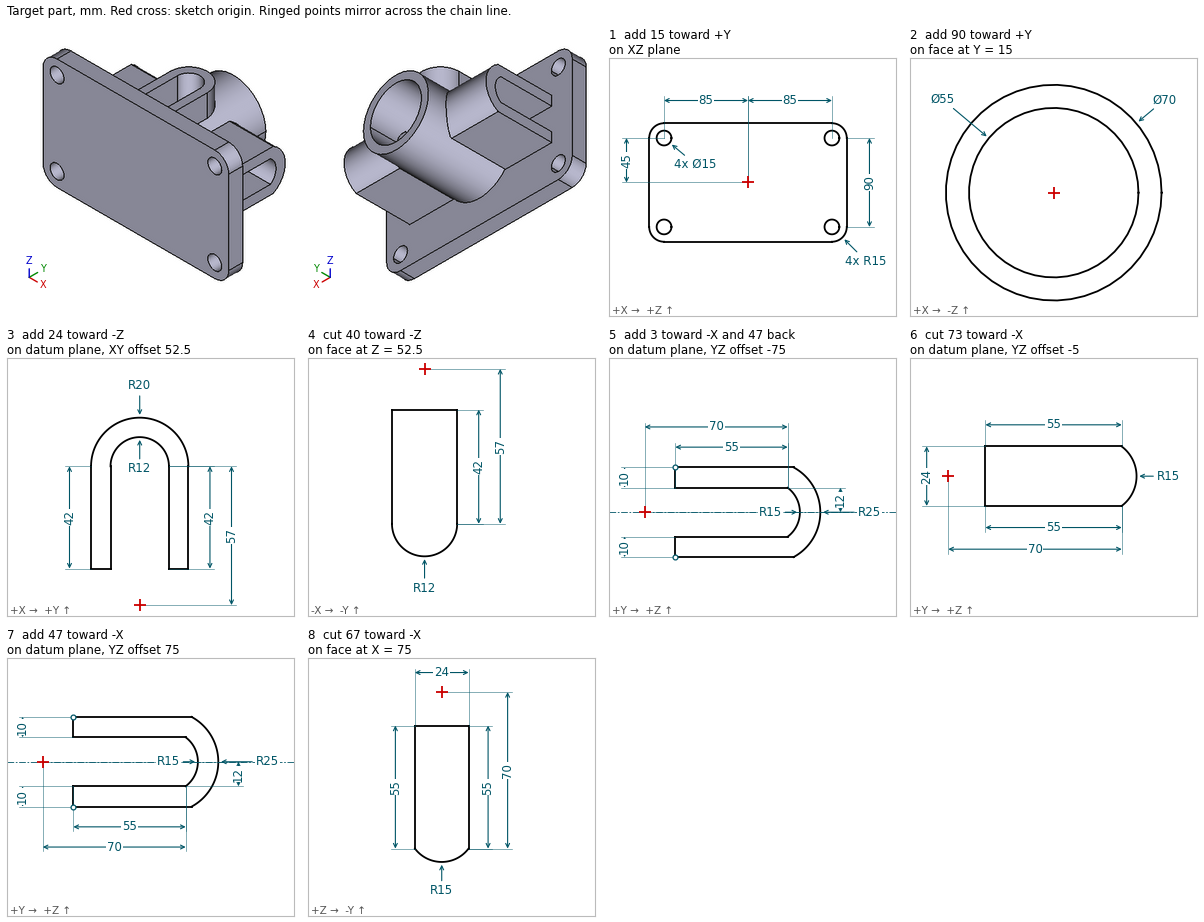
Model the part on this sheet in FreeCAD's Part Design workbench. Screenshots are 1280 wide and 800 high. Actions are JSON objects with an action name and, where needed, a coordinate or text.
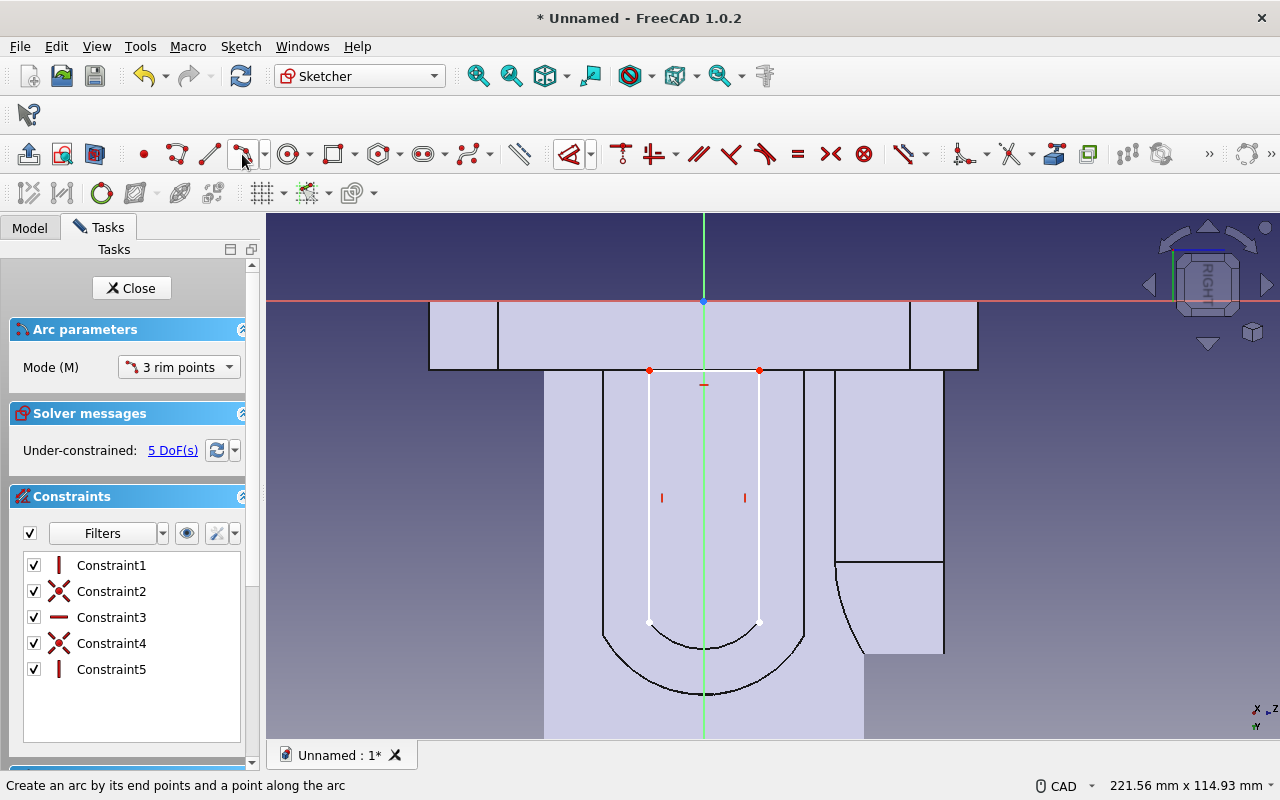
{"action": "left_click", "coordinate": [649, 623]}
{"action": "left_click", "coordinate": [759, 623]}
{"action": "left_click", "coordinate": [679, 645]}
{"action": "key", "text": "Escape"}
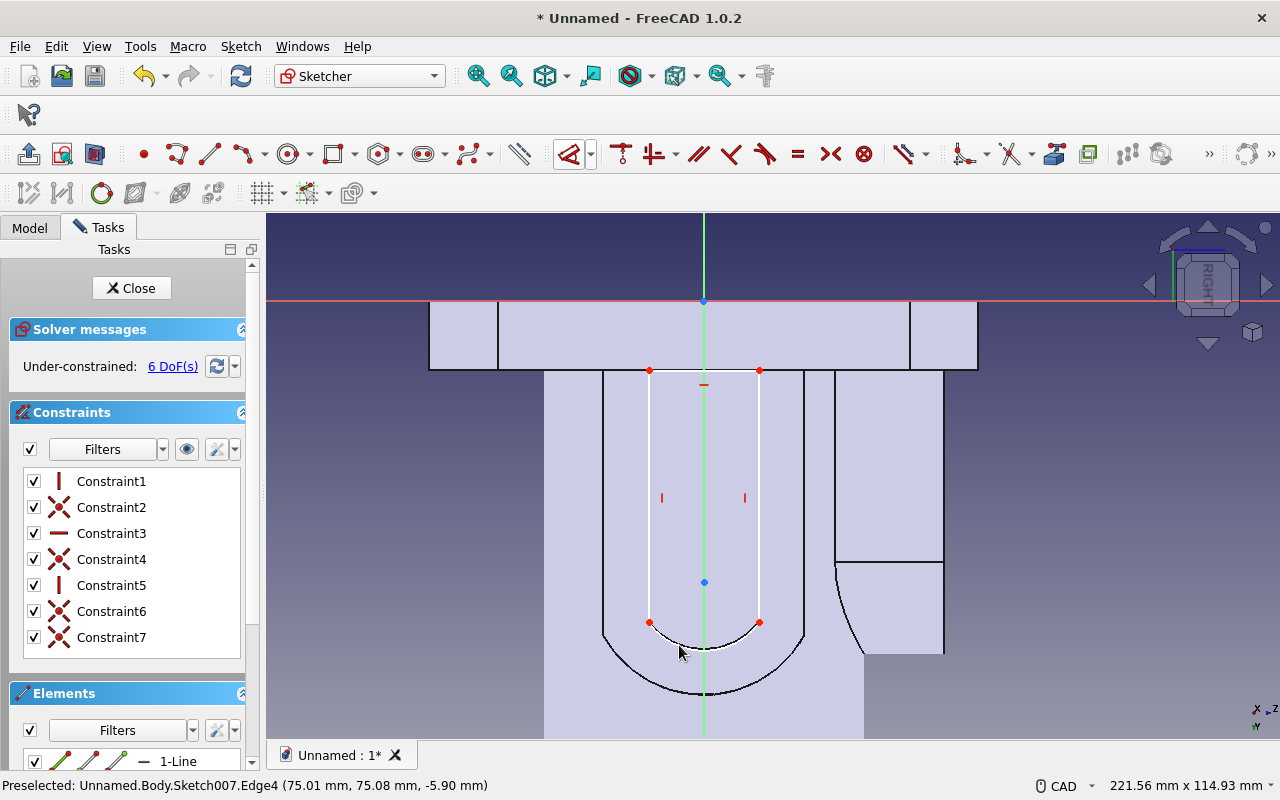
{"action": "left_click", "coordinate": [704, 582]}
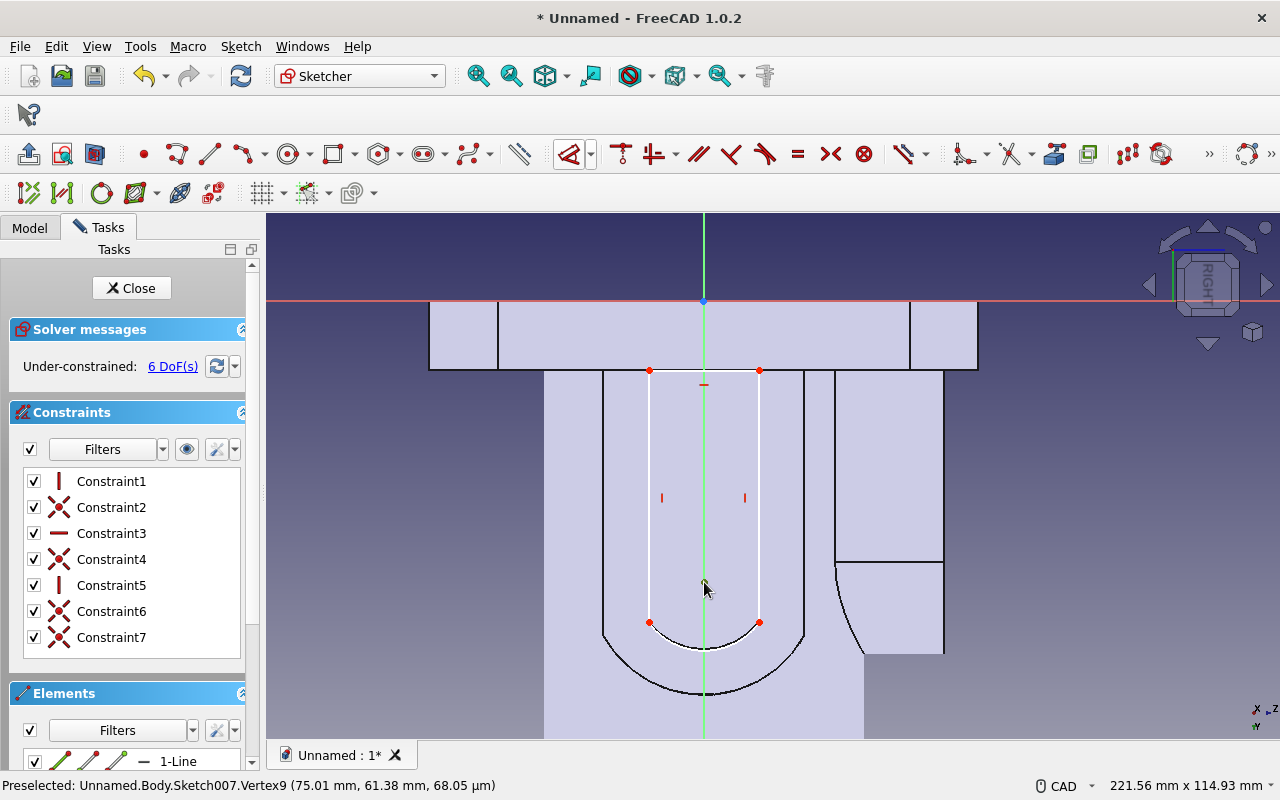
{"action": "left_click", "coordinate": [704, 610]}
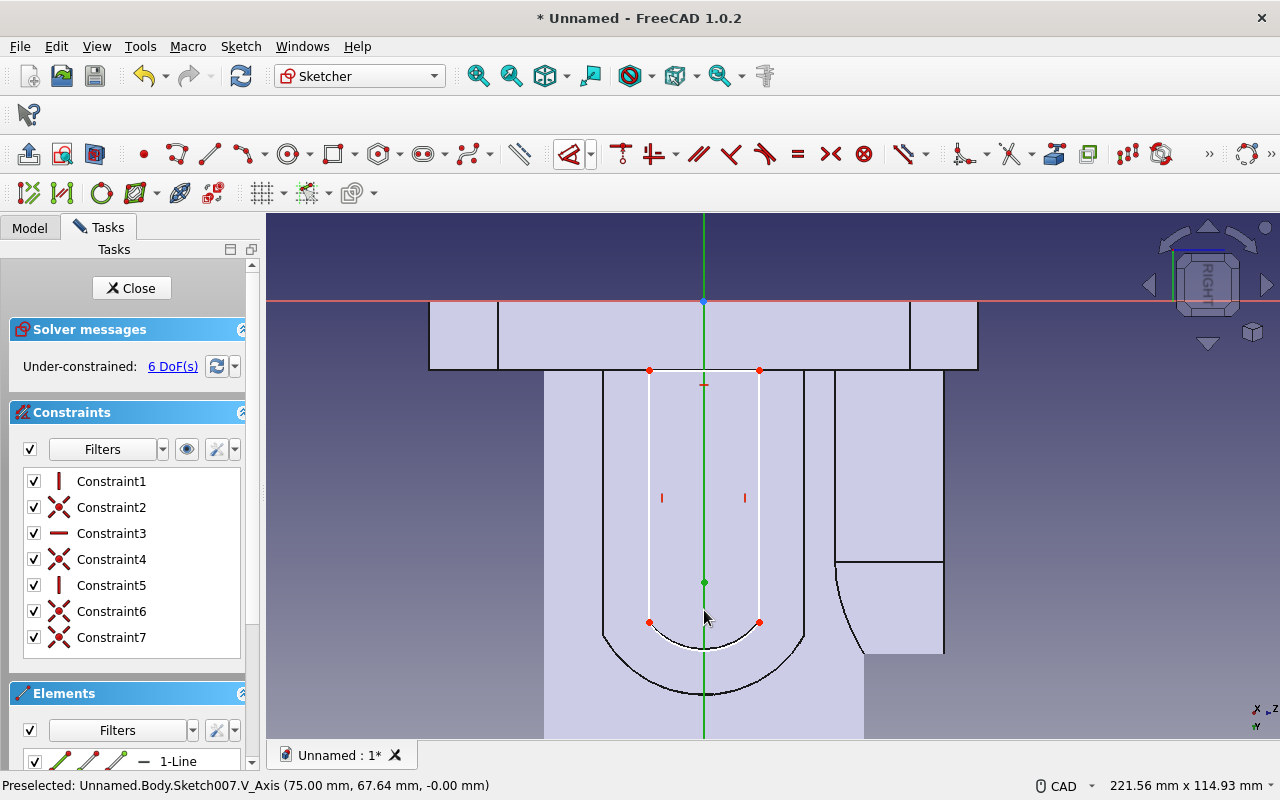
{"action": "key", "text": "c"}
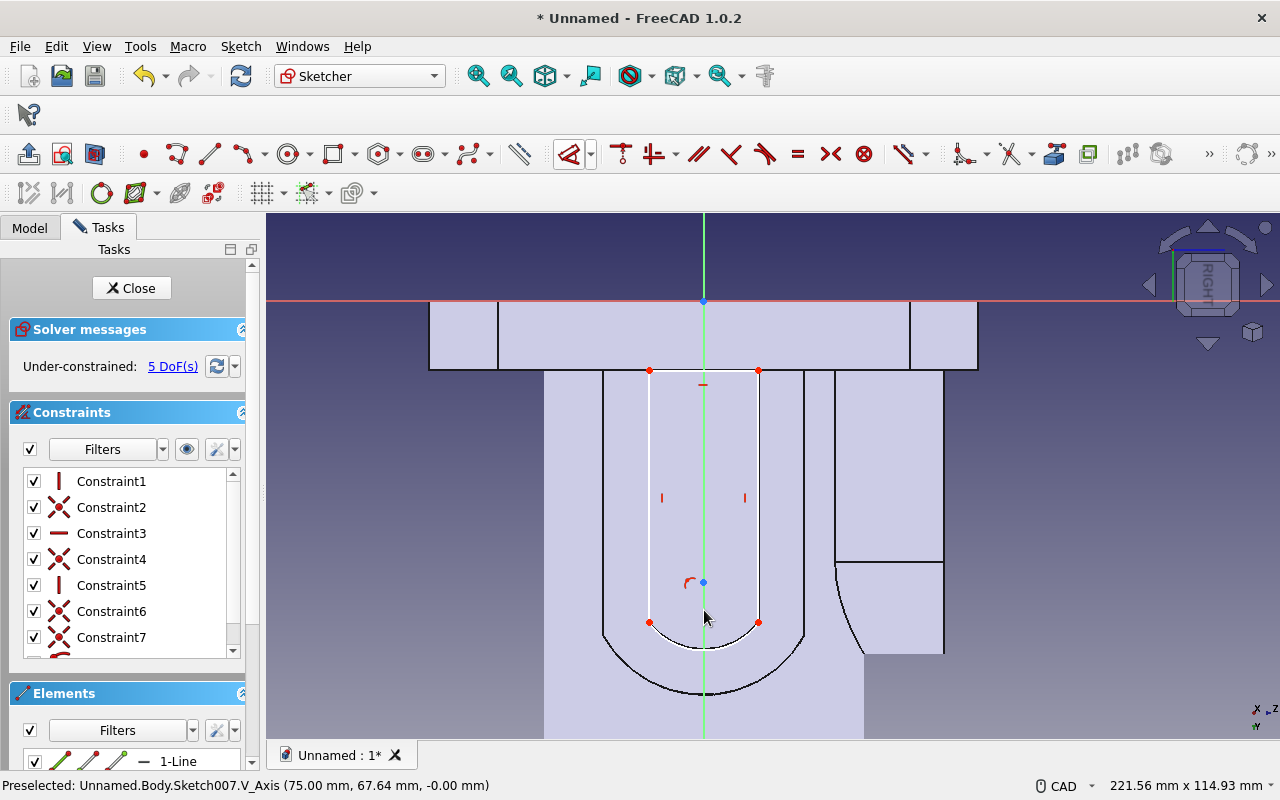
{"action": "left_click", "coordinate": [679, 646]}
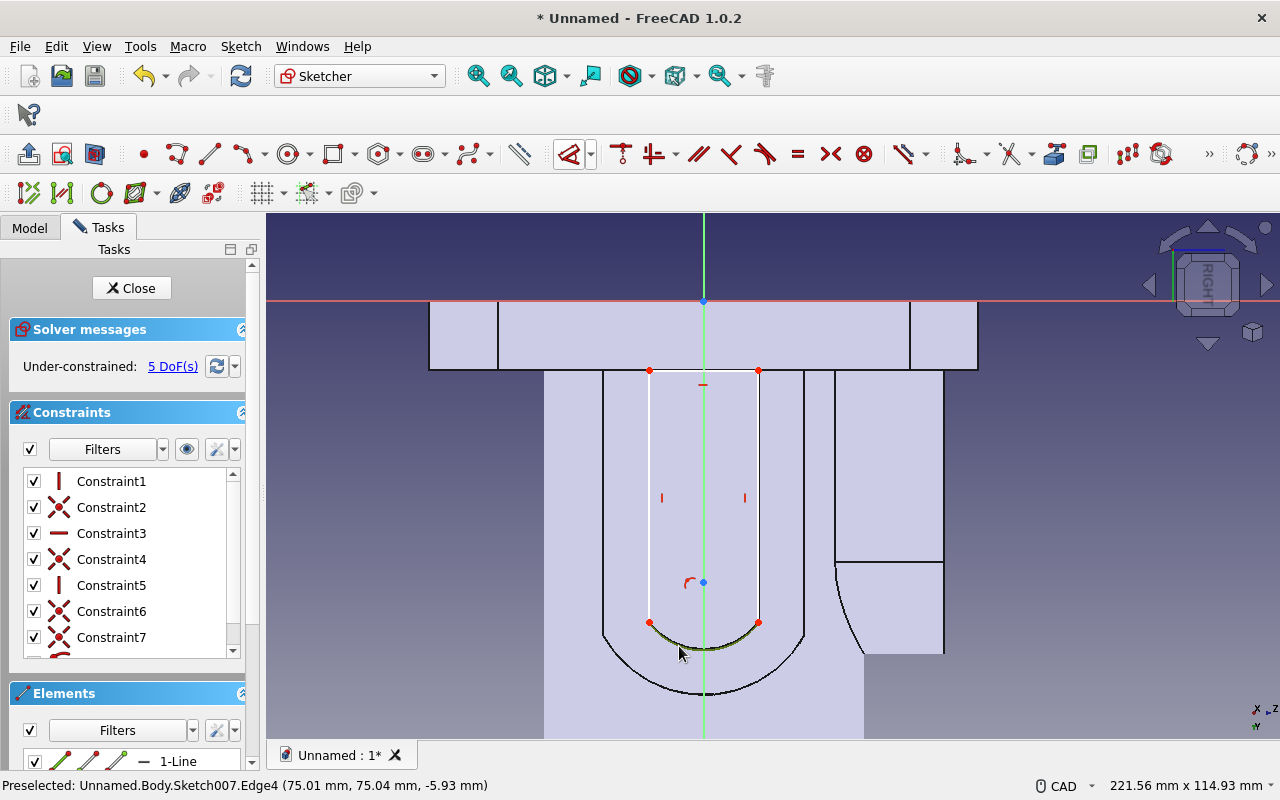
{"action": "key", "text": "k r"}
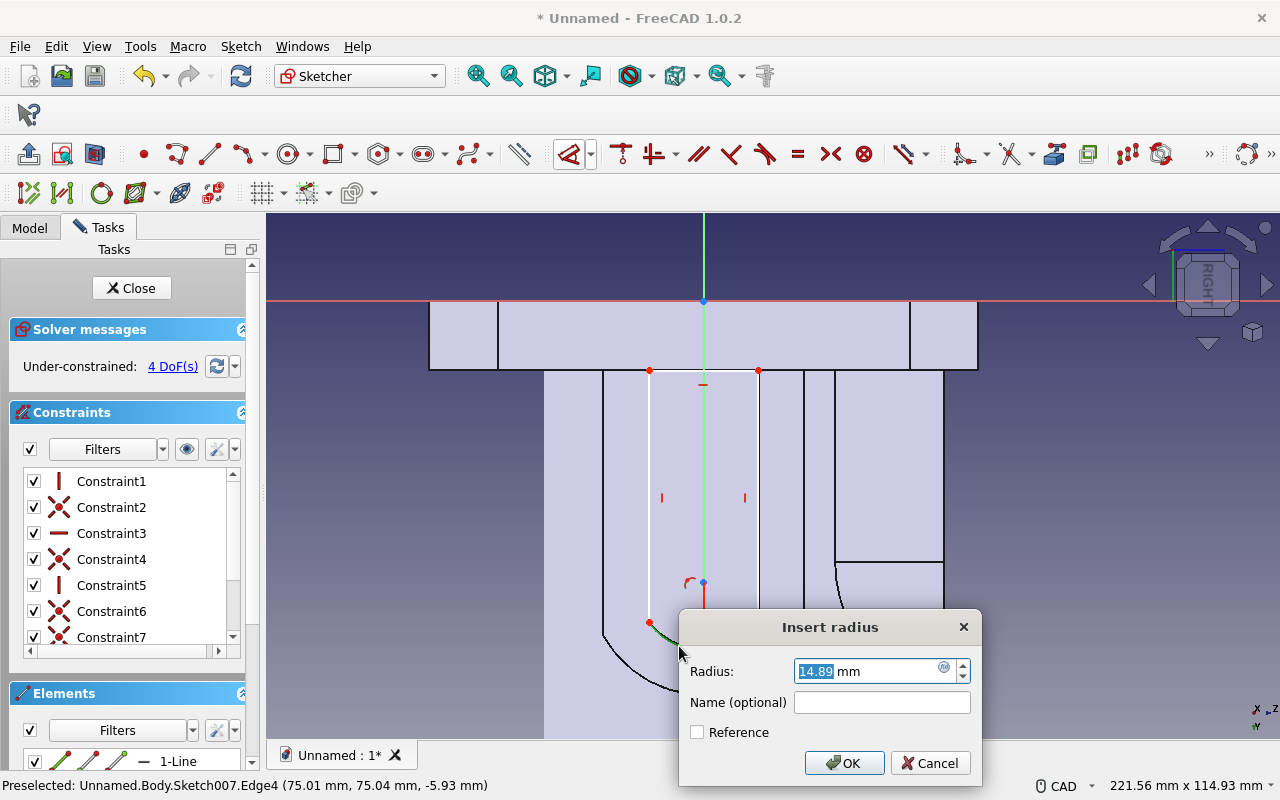
{"action": "type", "text": "15"}
{"action": "key", "text": "Return"}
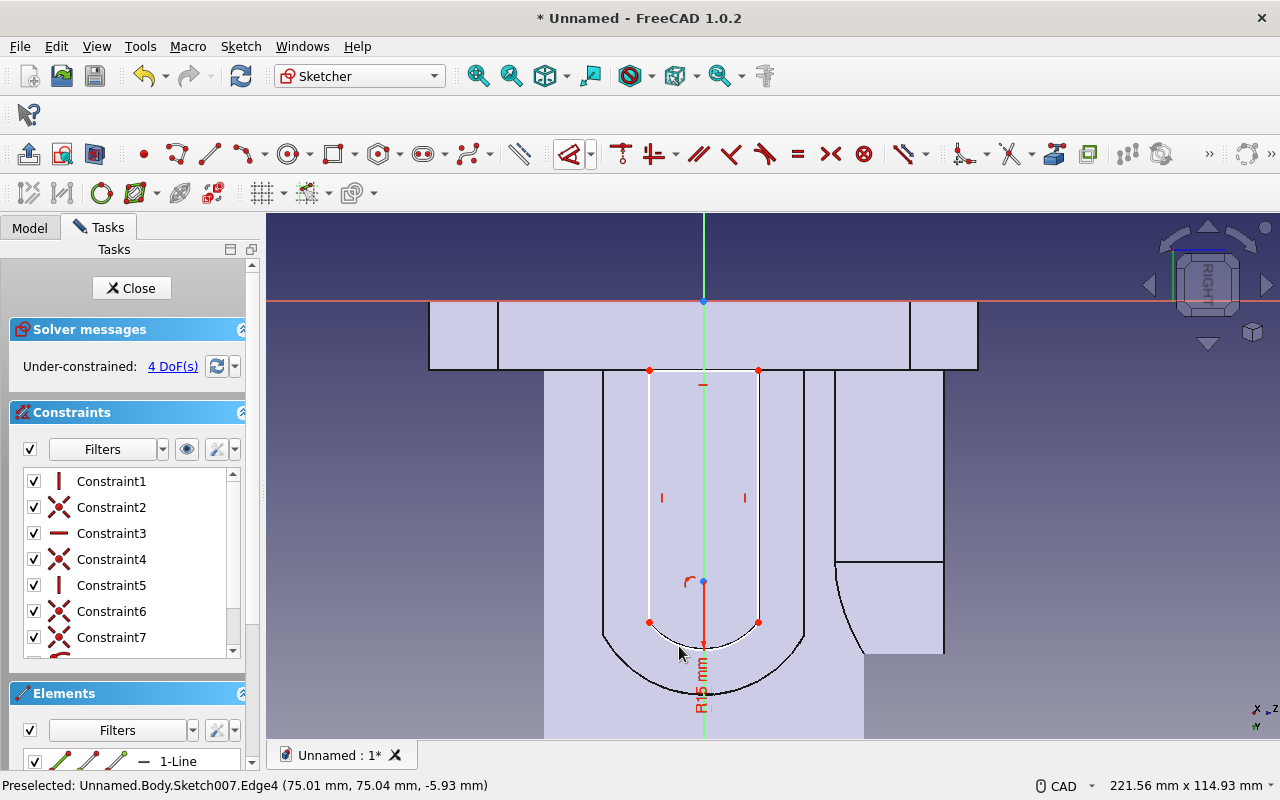
{"action": "left_click", "coordinate": [758, 547]}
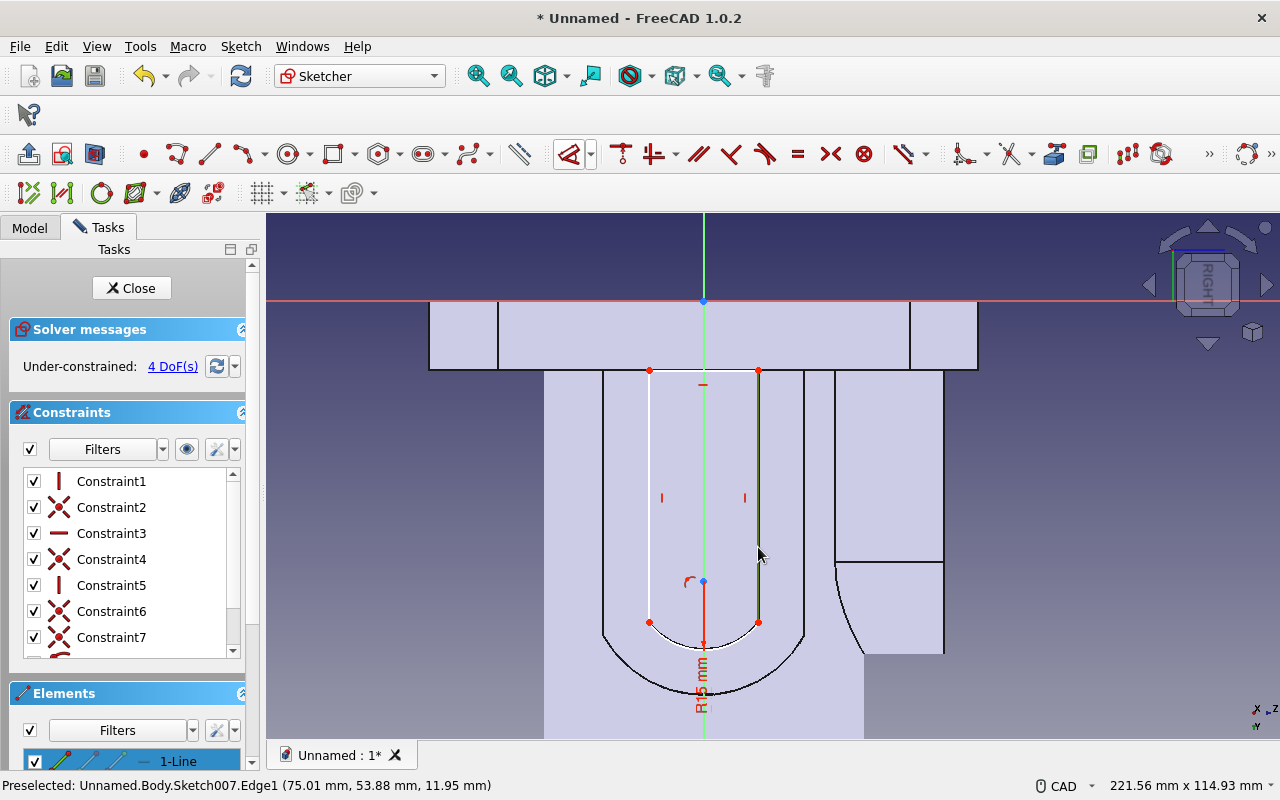
{"action": "key", "text": "i"}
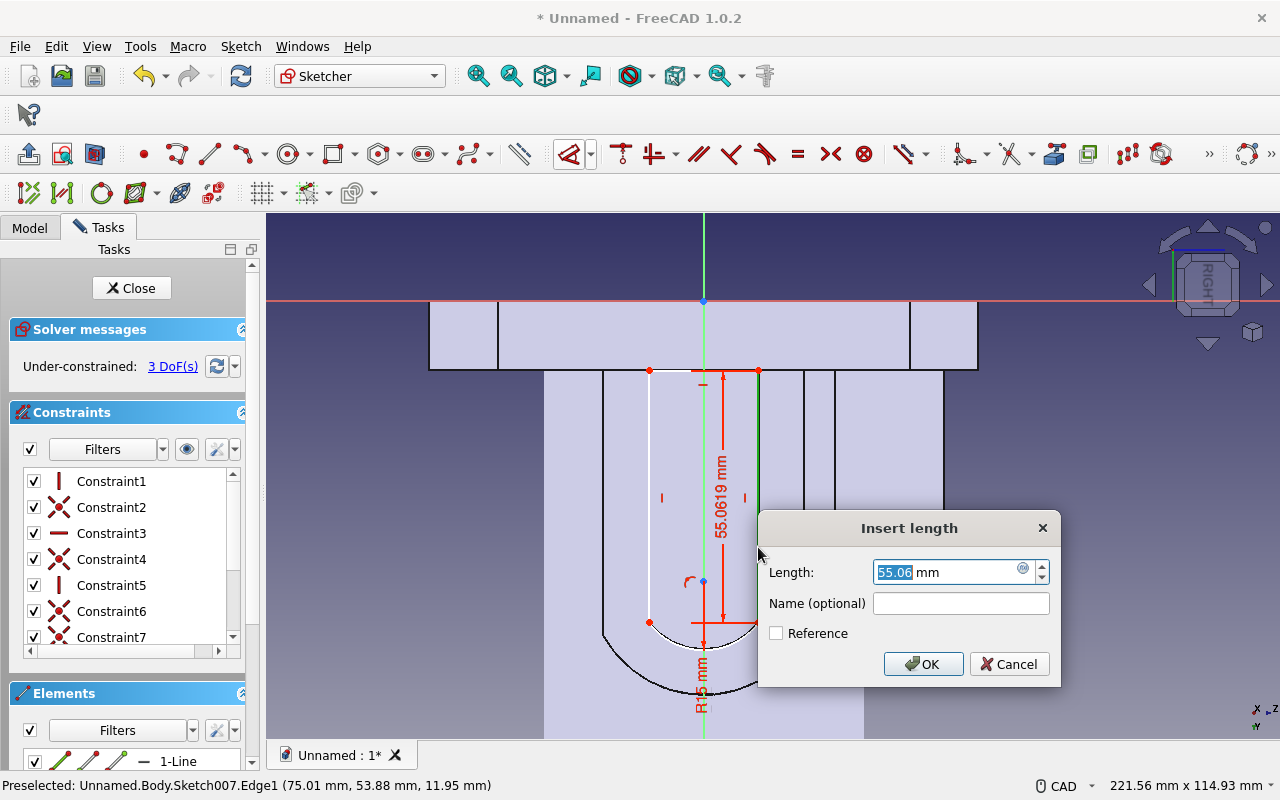
{"action": "type", "text": "55"}
{"action": "key", "text": "Return"}